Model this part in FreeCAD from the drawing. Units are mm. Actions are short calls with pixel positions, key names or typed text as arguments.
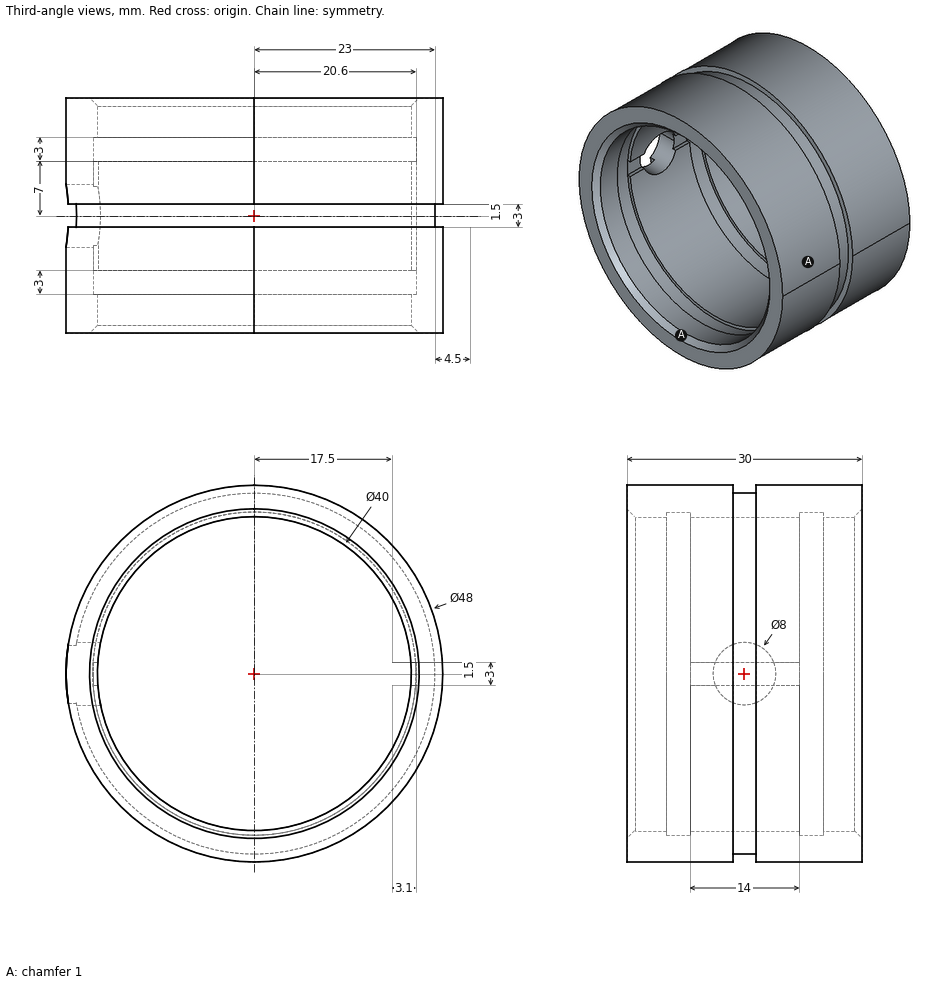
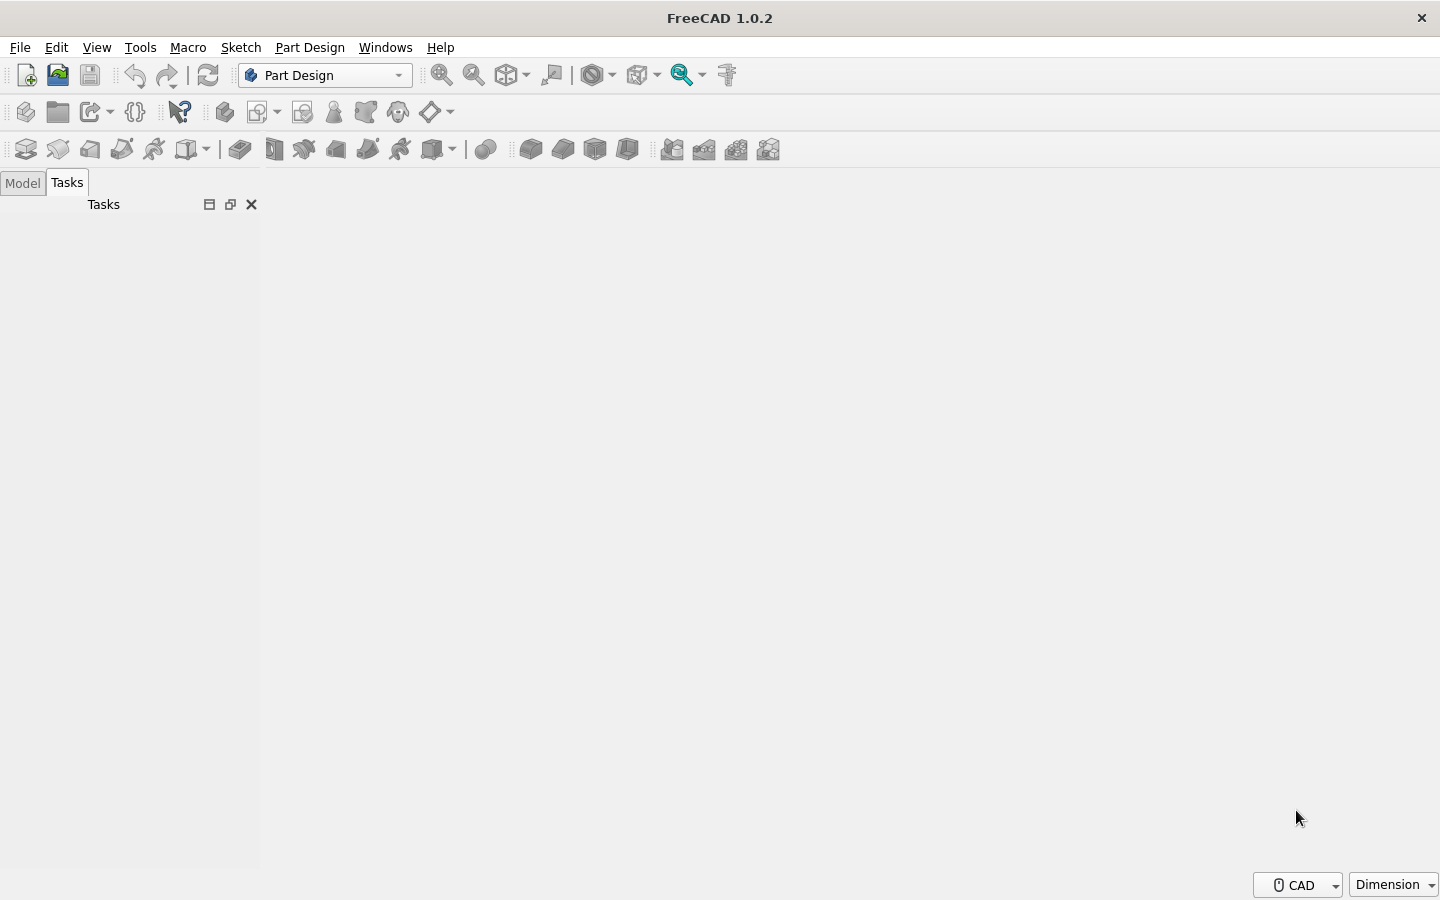
click(168, 76)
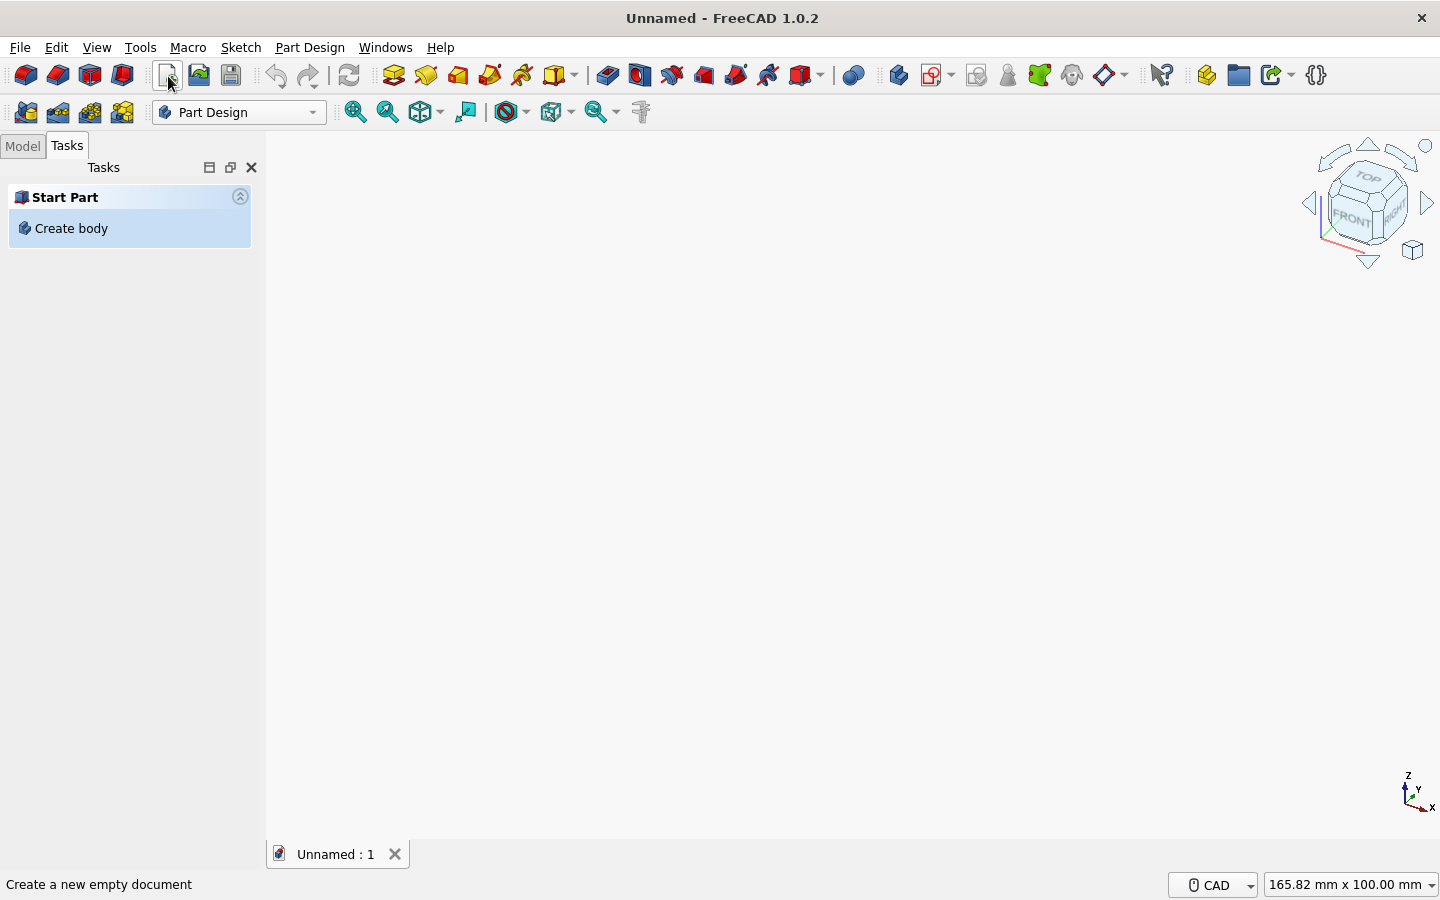
click(932, 76)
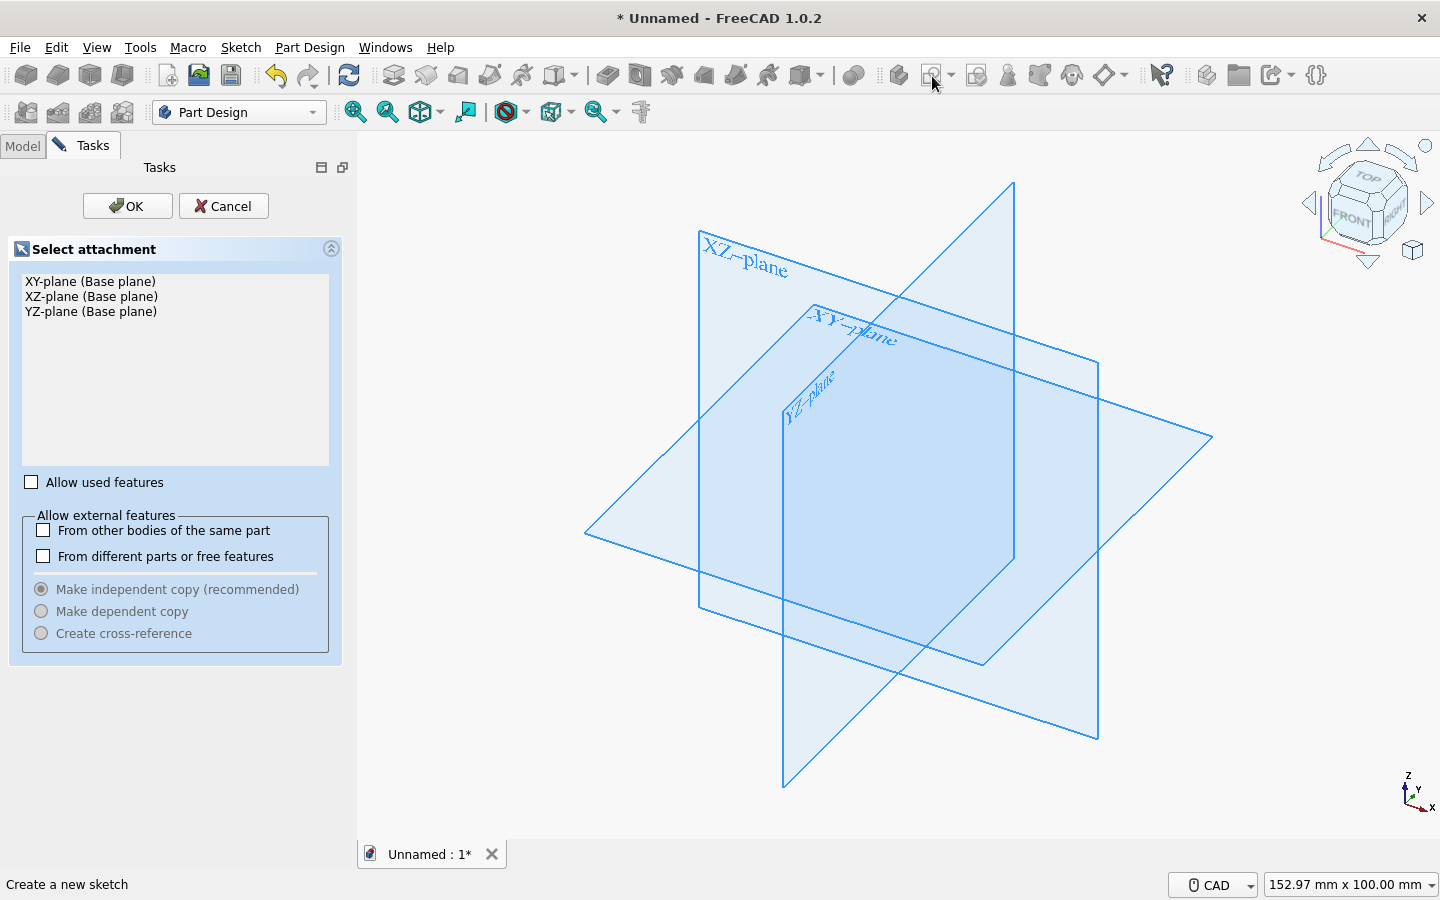
click(82, 296)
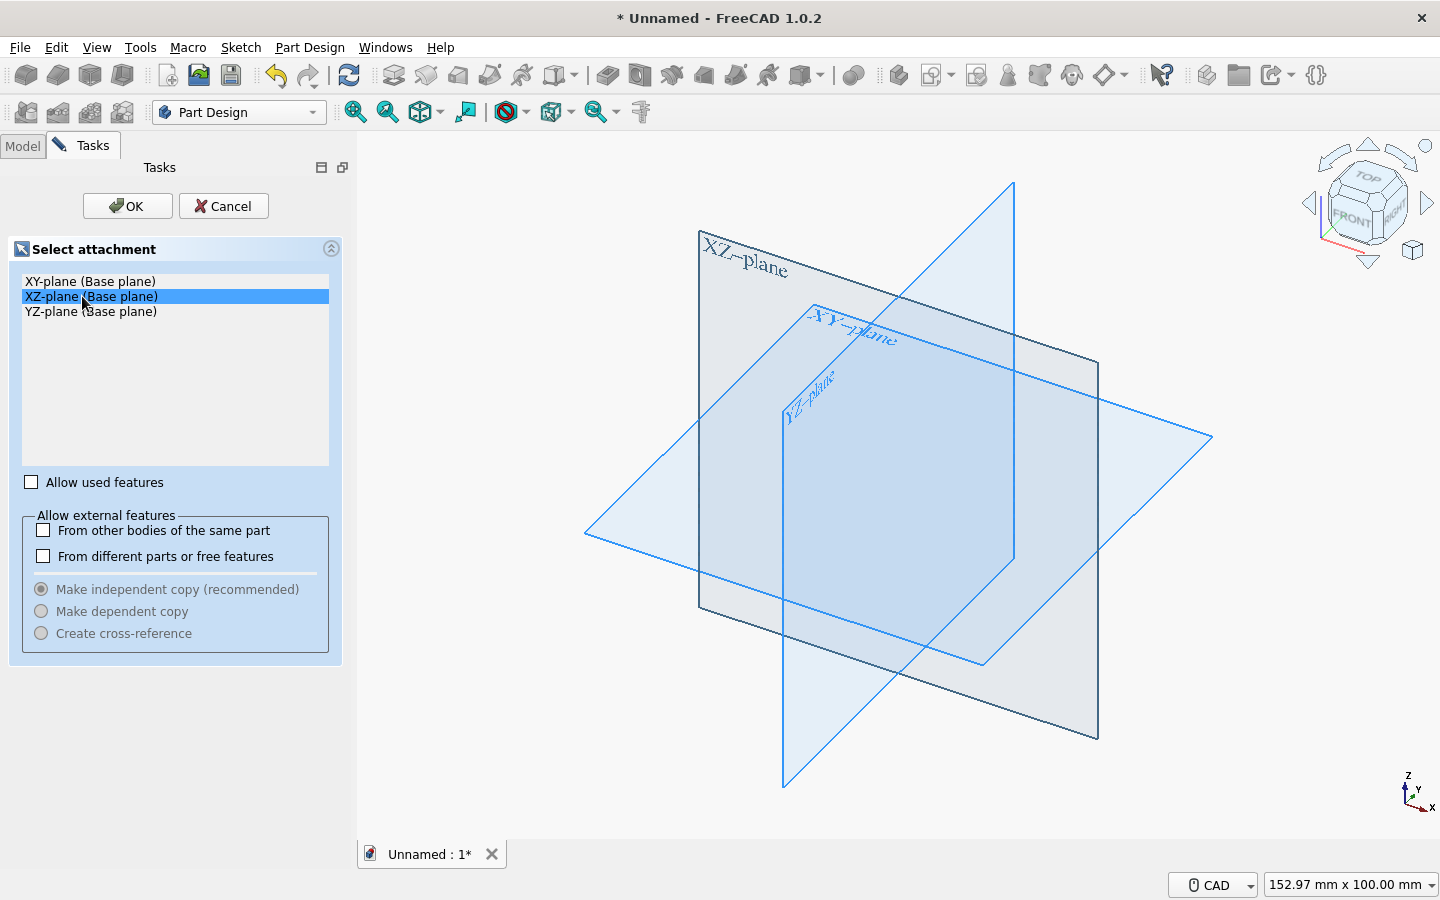
click(128, 206)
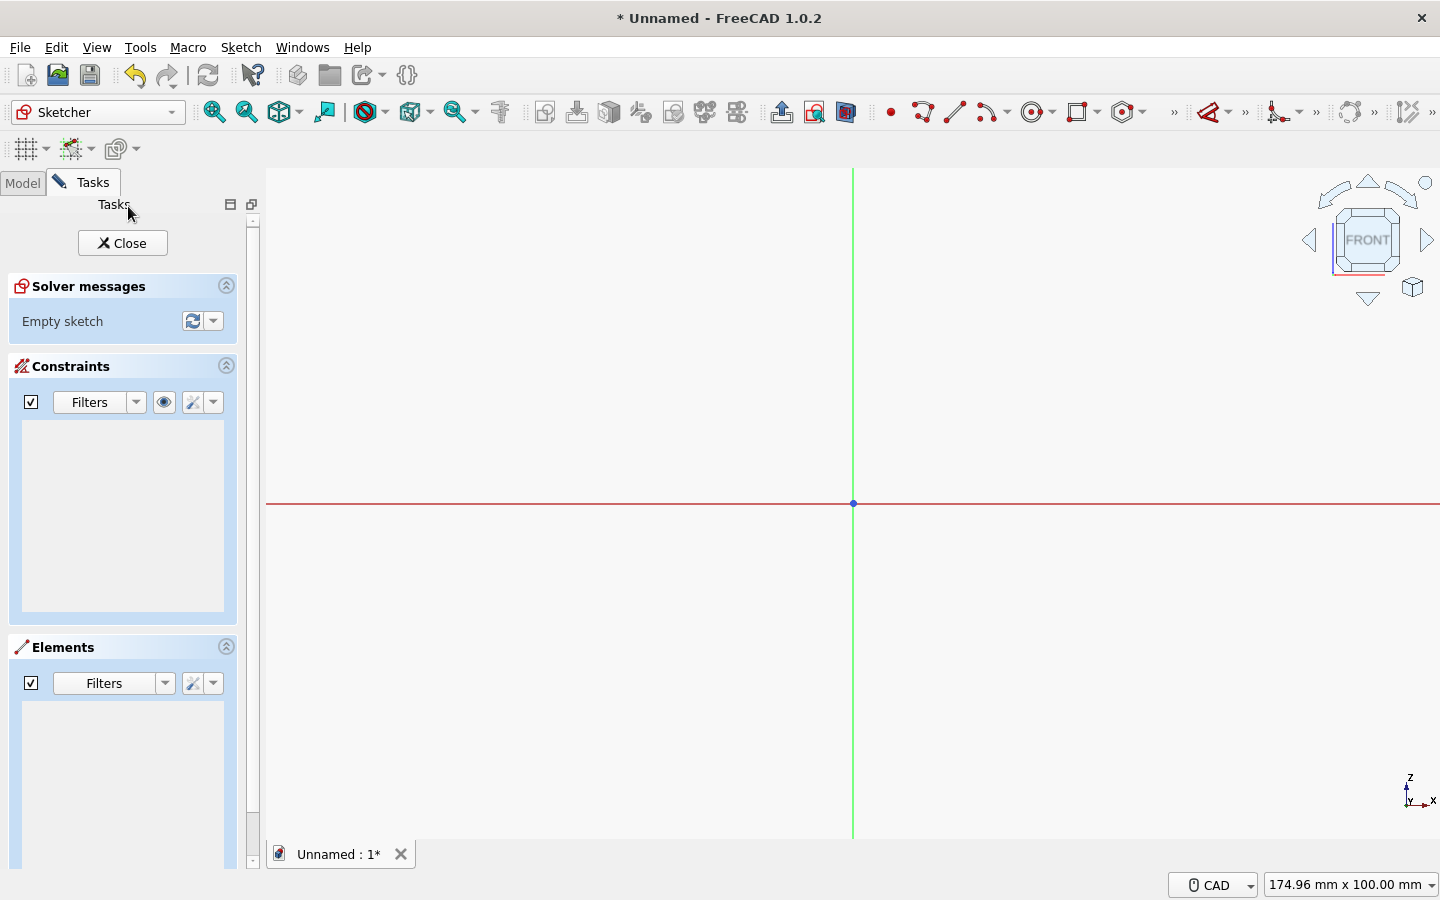
click(1032, 112)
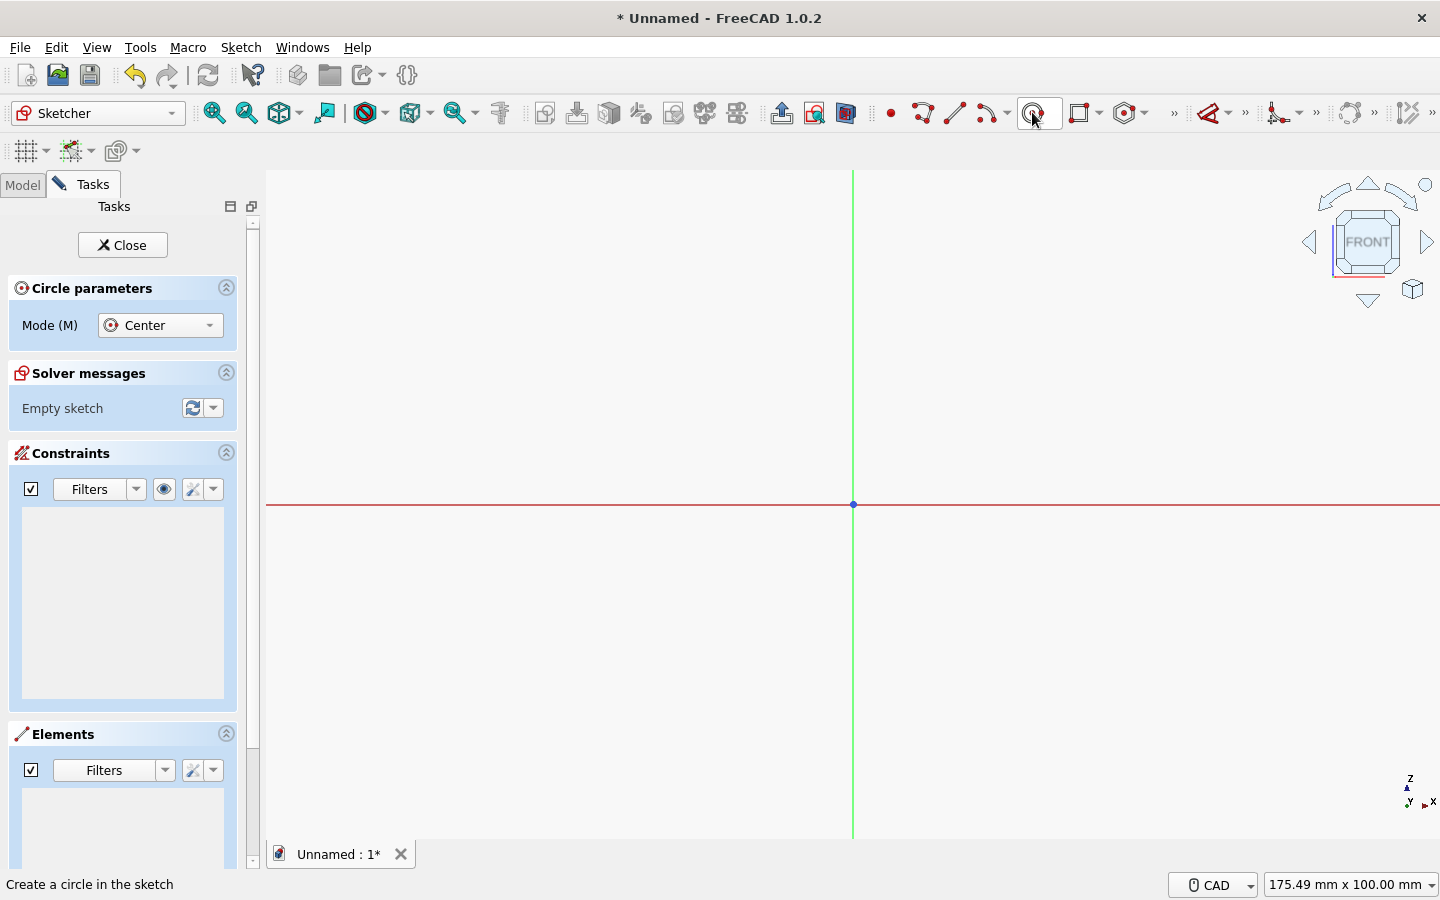
click(853, 504)
click(967, 391)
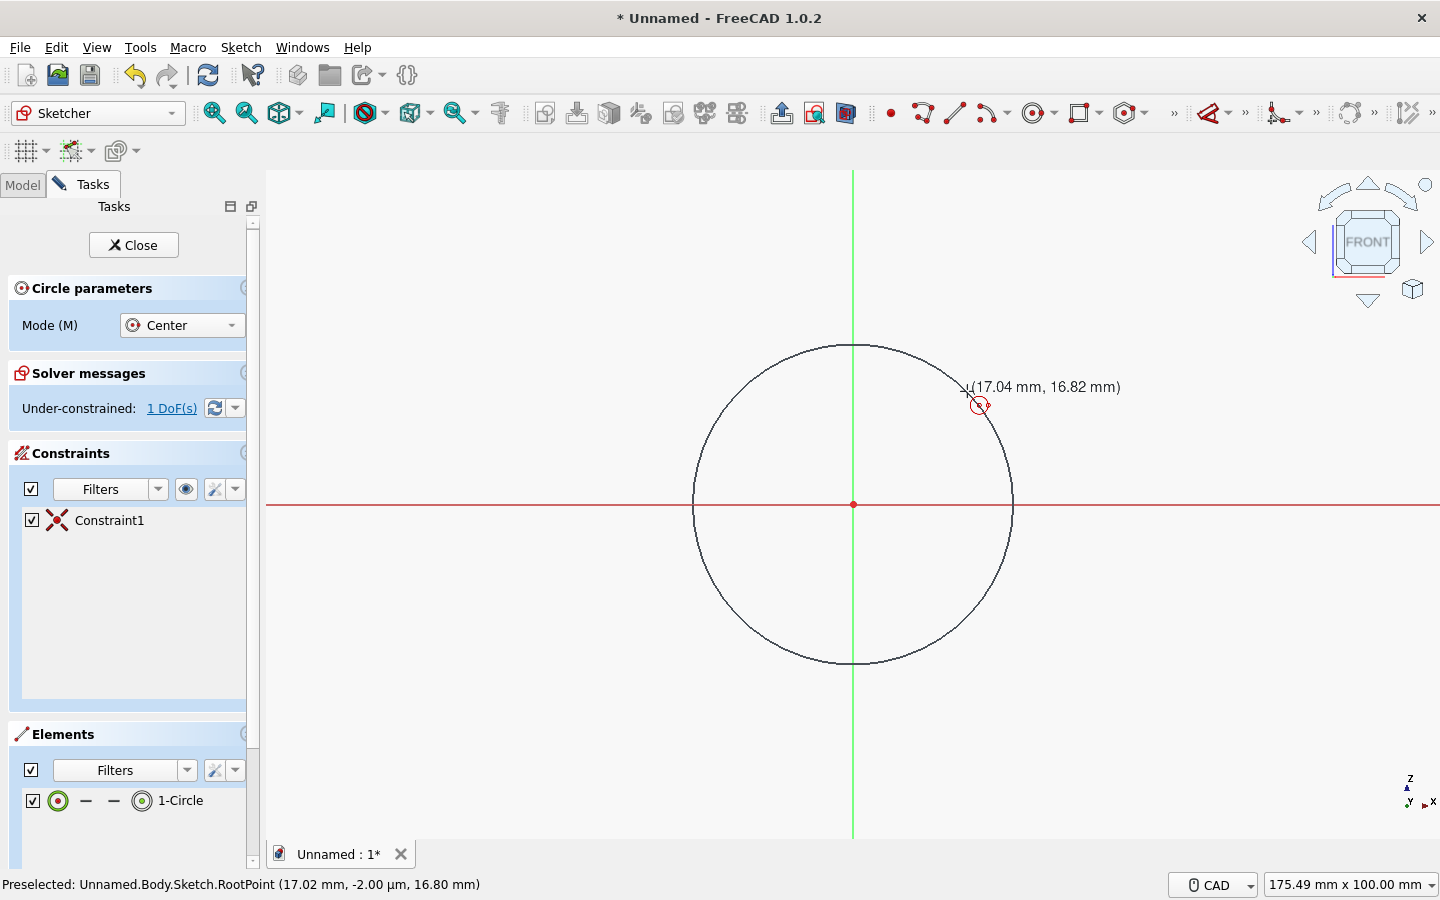
click(853, 504)
click(948, 410)
key(Escape)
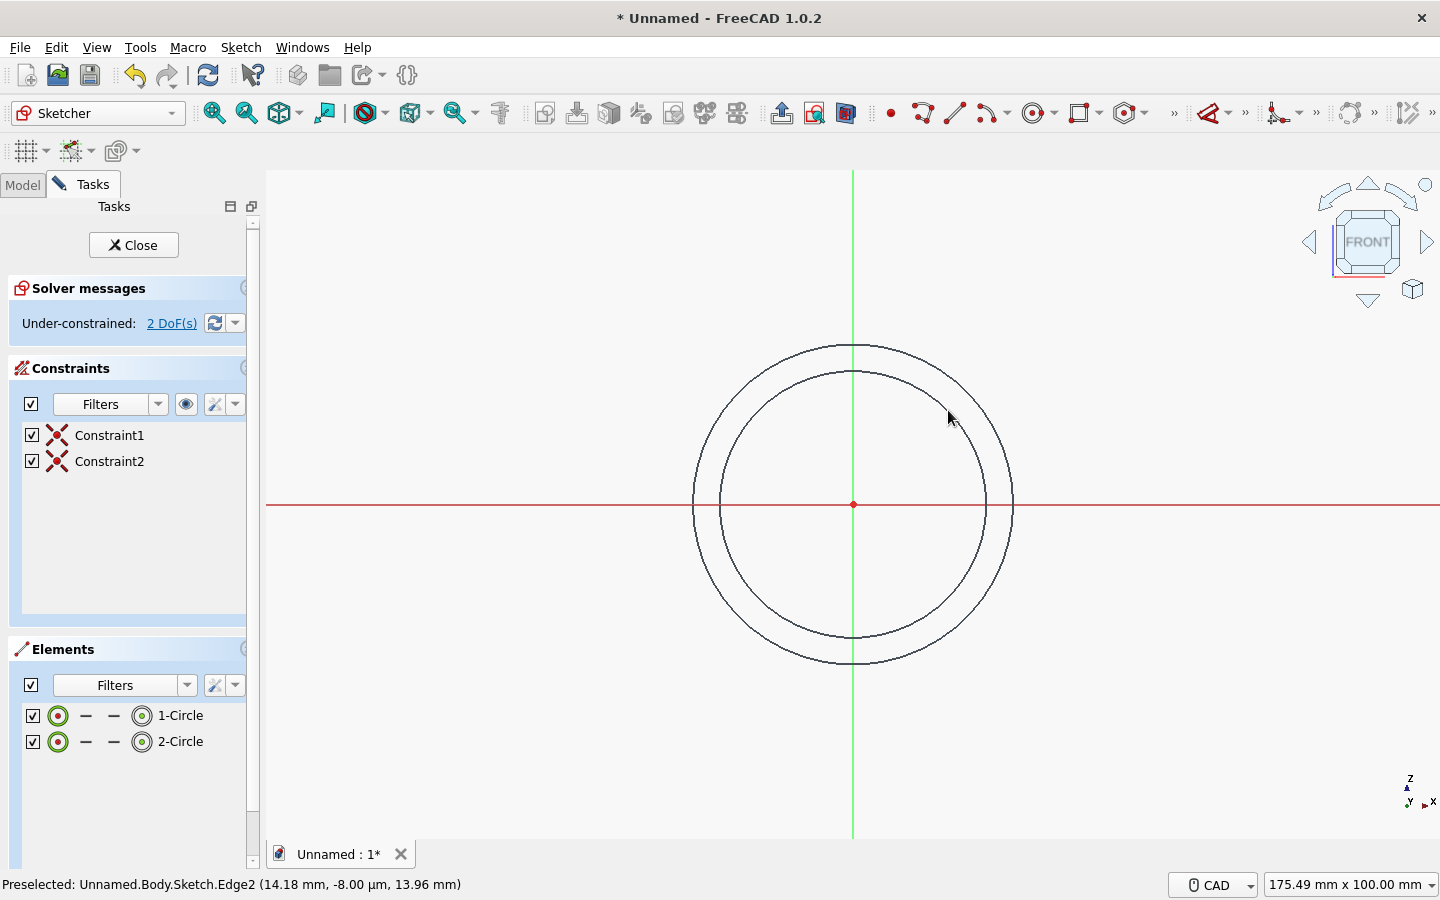
click(1208, 114)